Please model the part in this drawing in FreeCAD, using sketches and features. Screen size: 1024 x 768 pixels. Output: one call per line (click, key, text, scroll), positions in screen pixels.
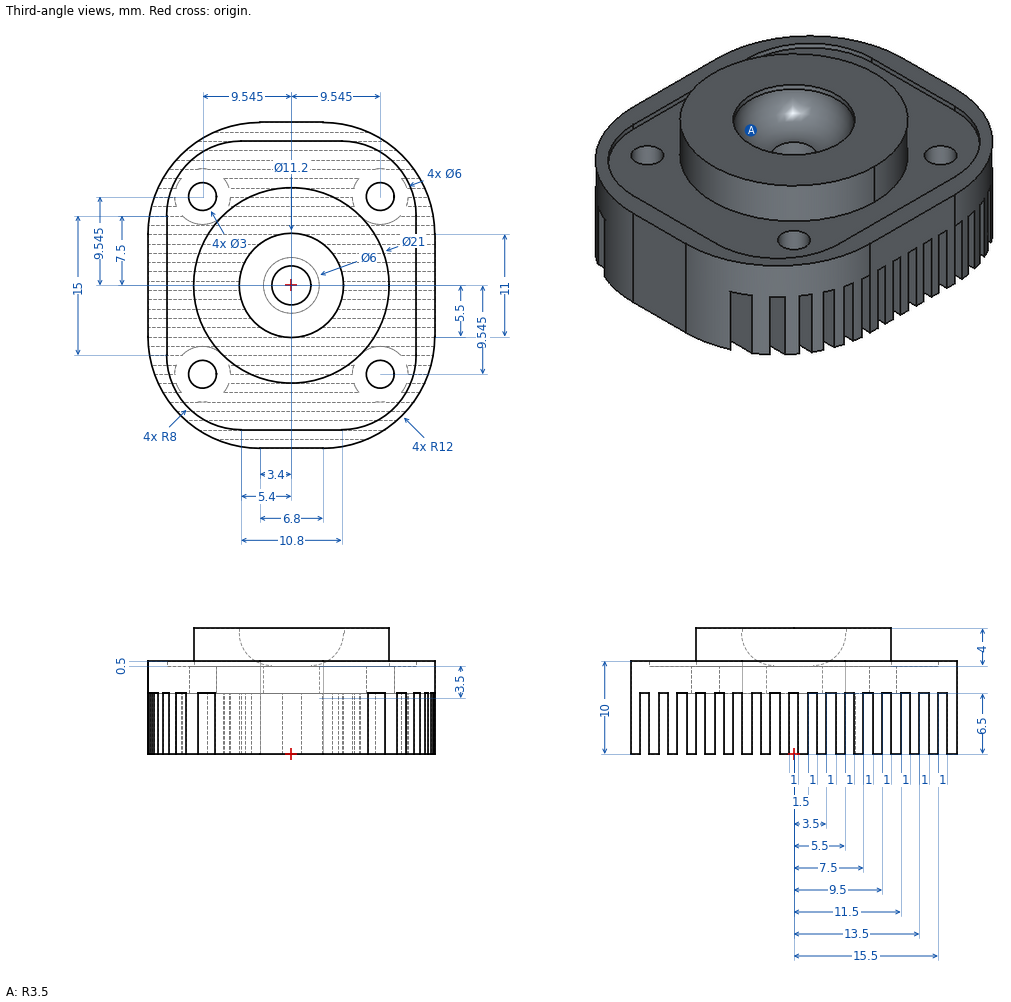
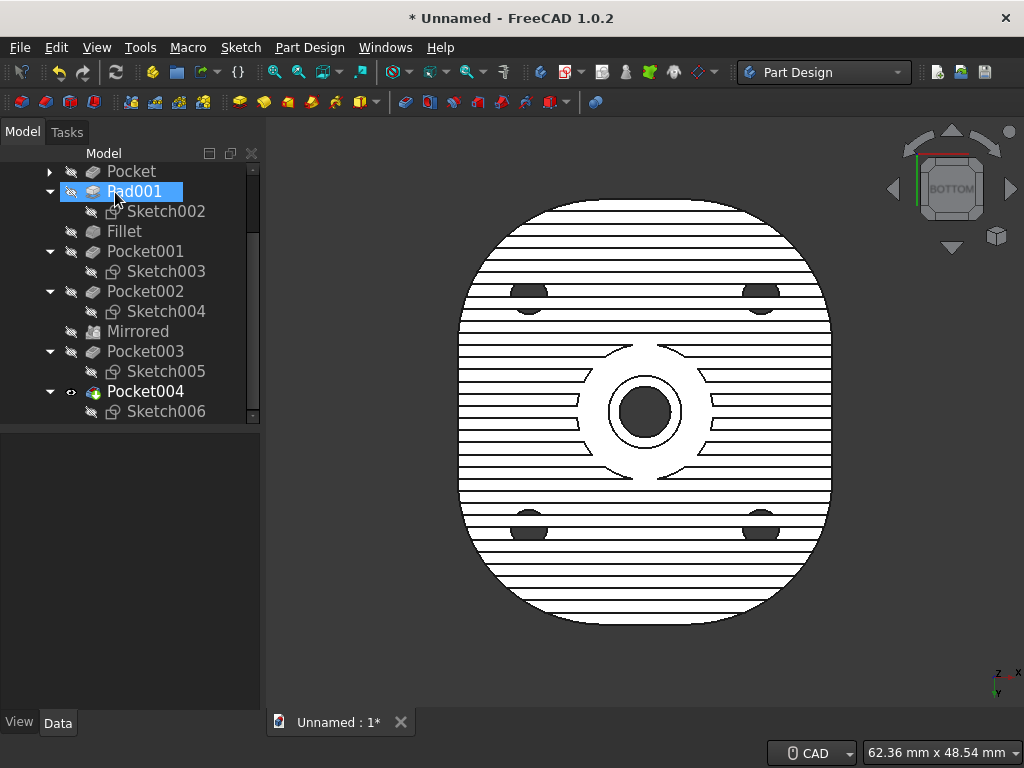
click(592, 411)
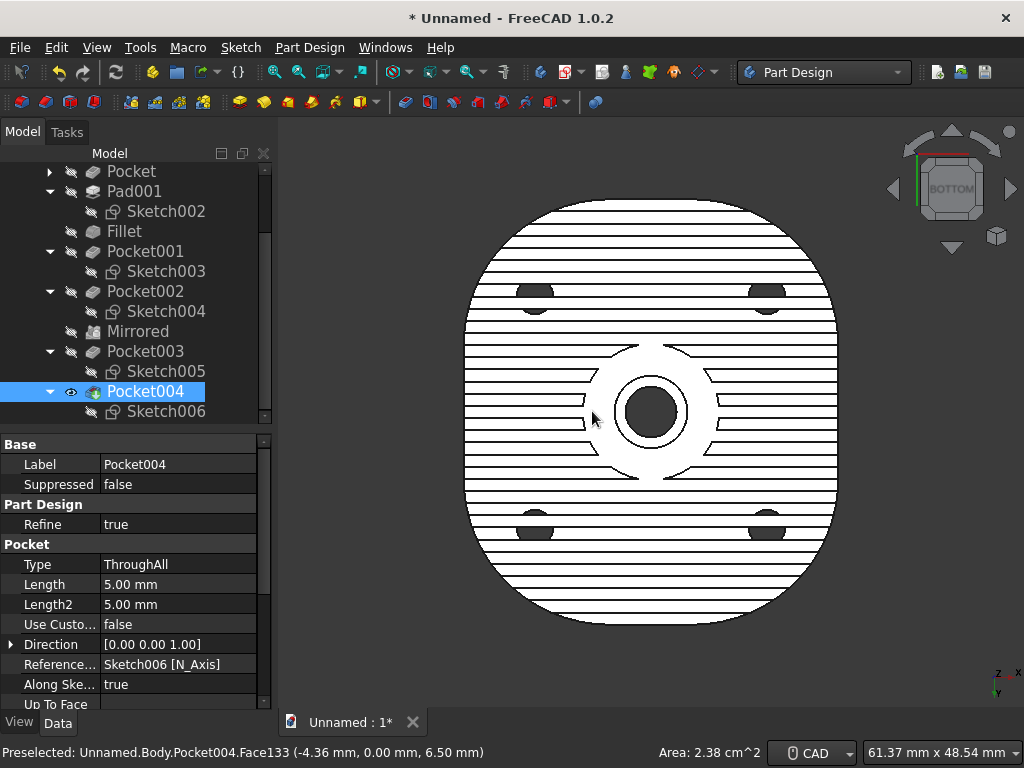
click(566, 72)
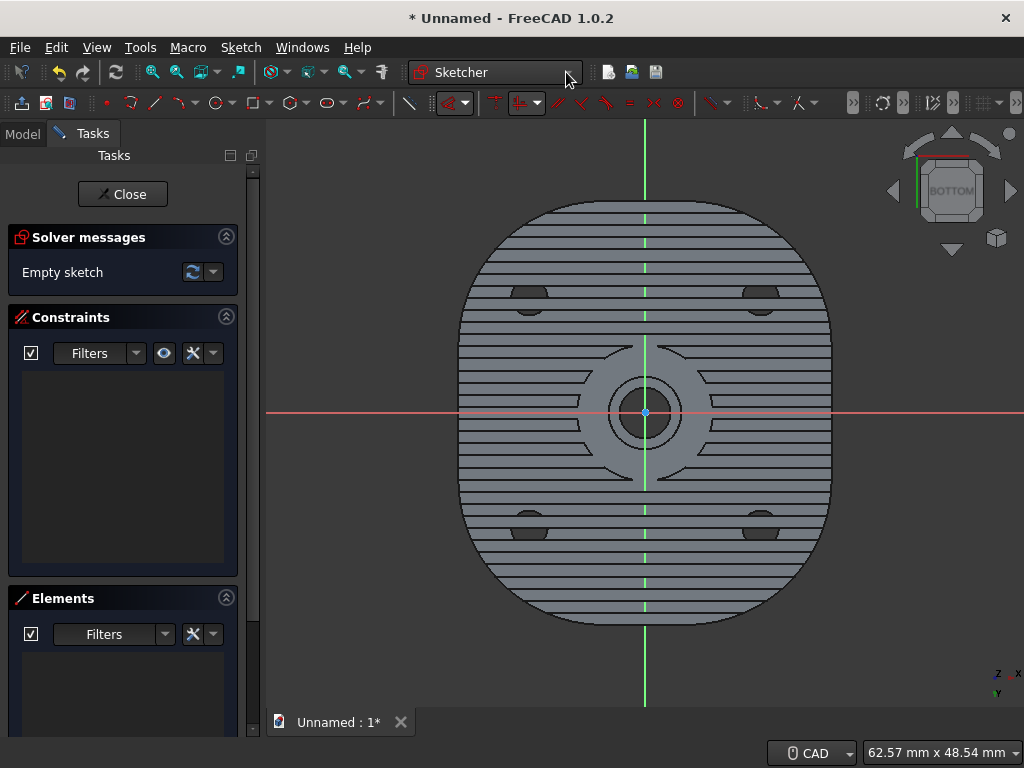
click(70, 104)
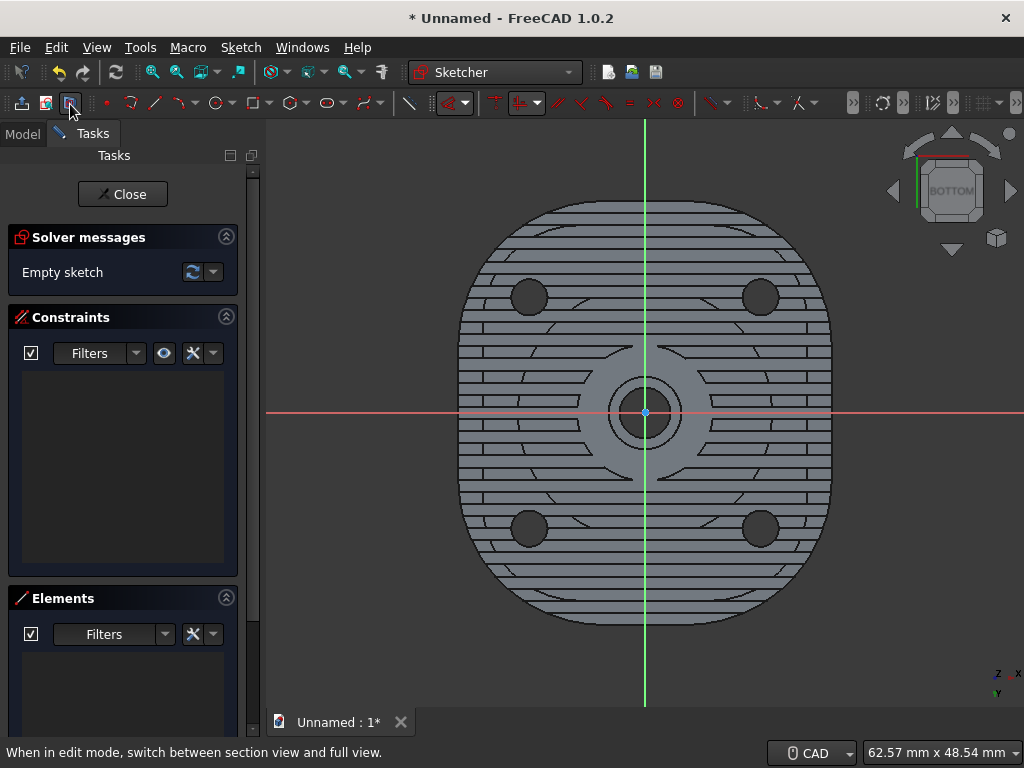
click(216, 104)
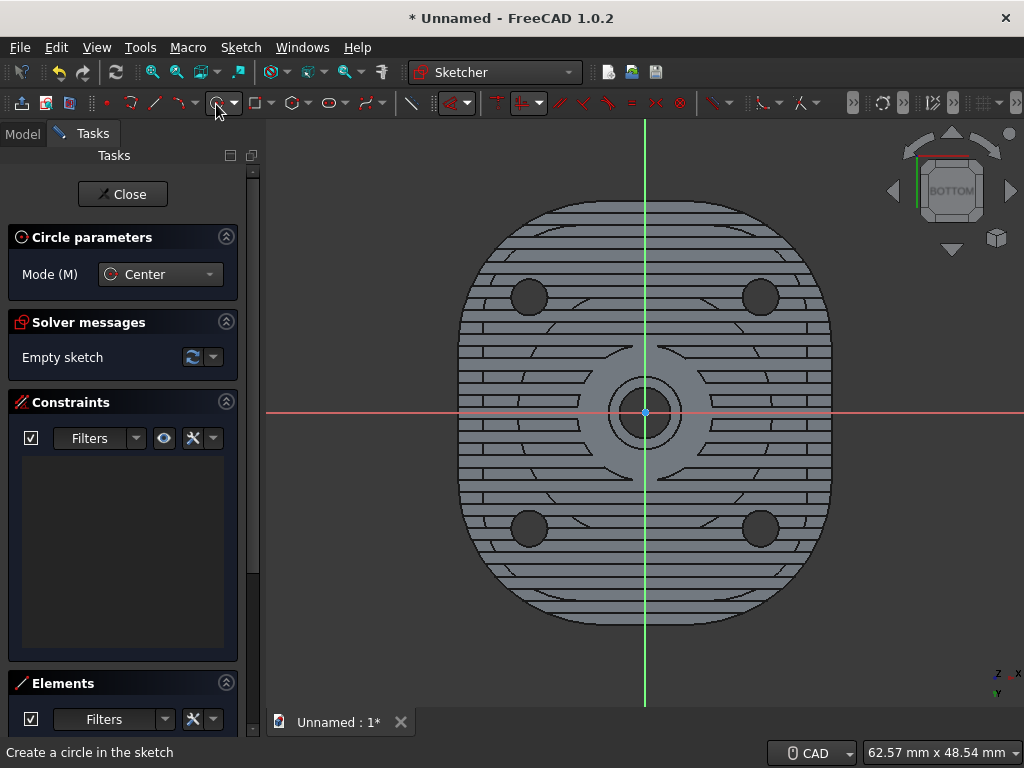
click(761, 529)
move(786, 503)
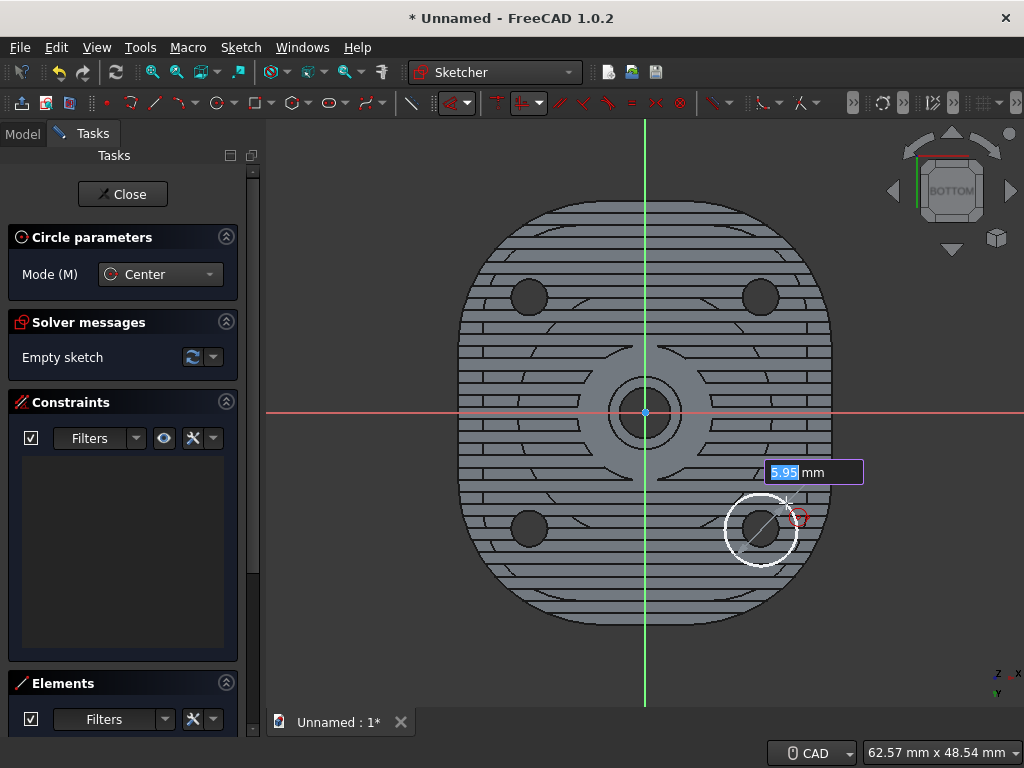
text(6)
key(Return)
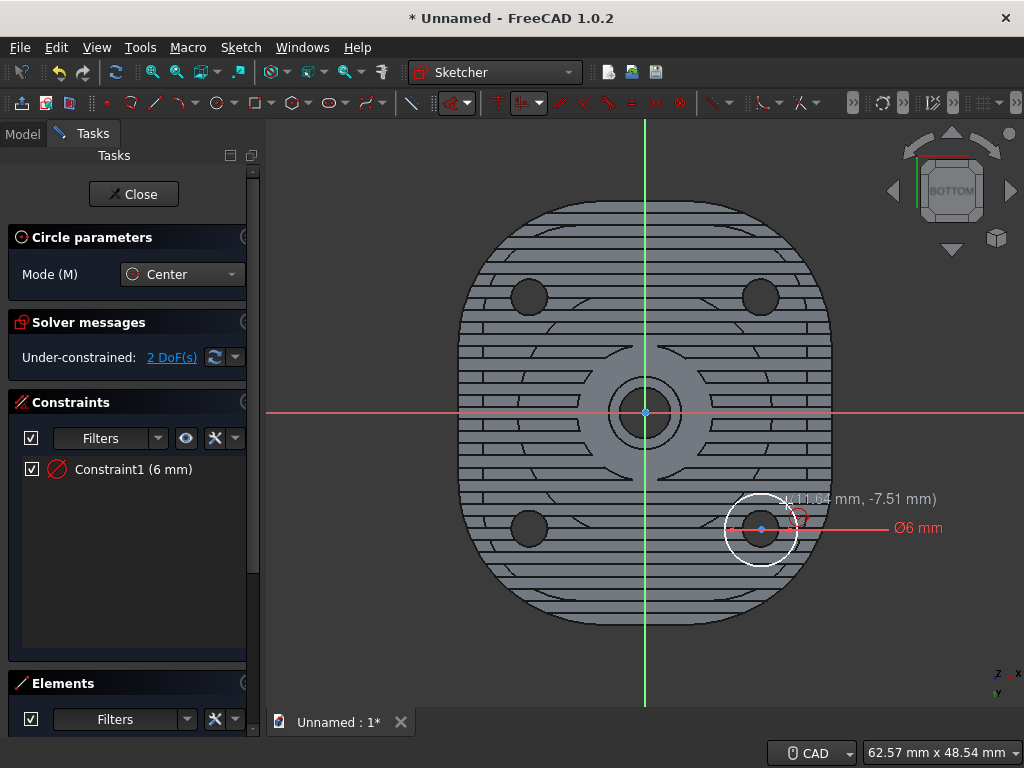
click(529, 529)
move(555, 503)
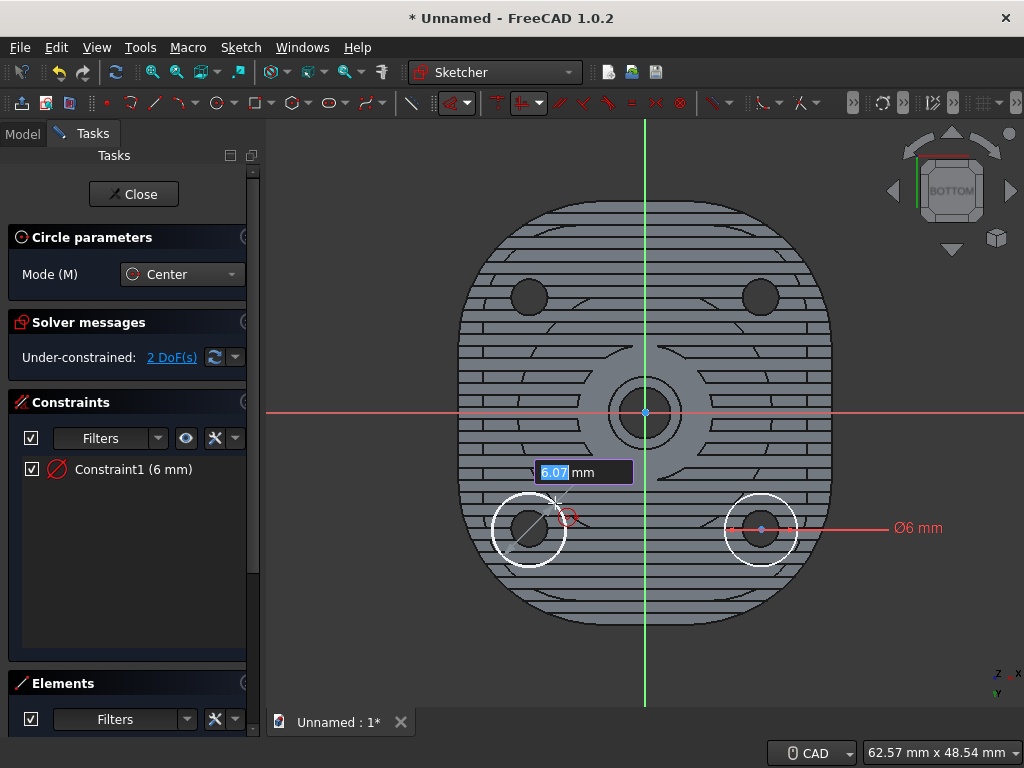
text(6)
key(Return)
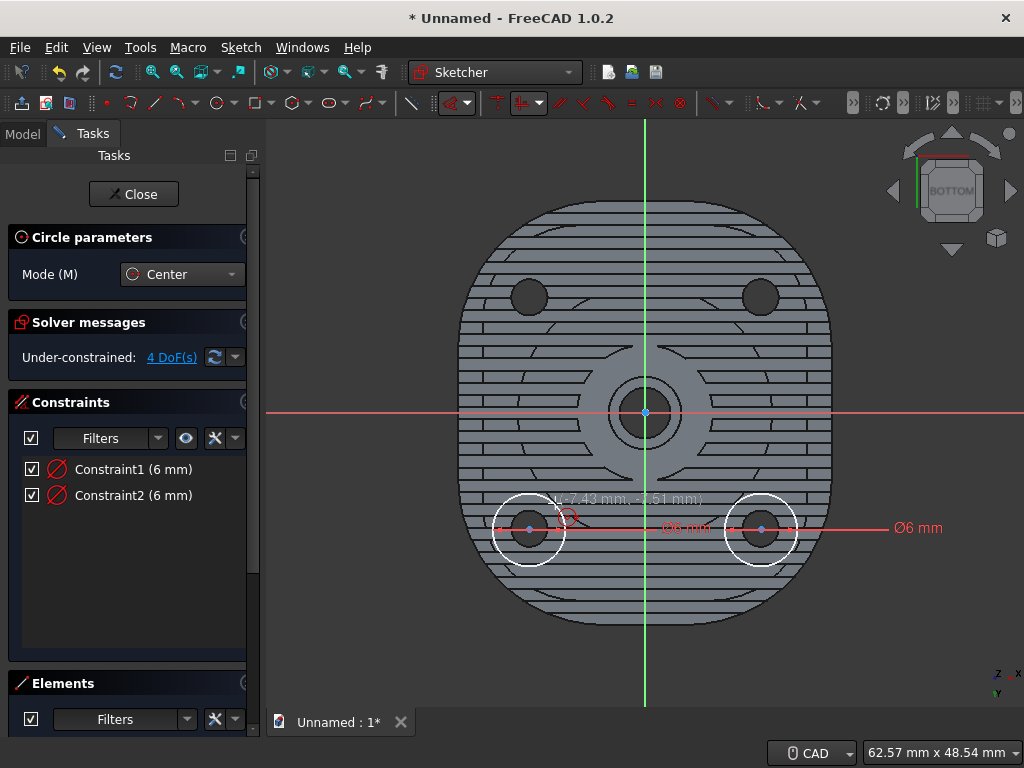
click(761, 297)
move(786, 272)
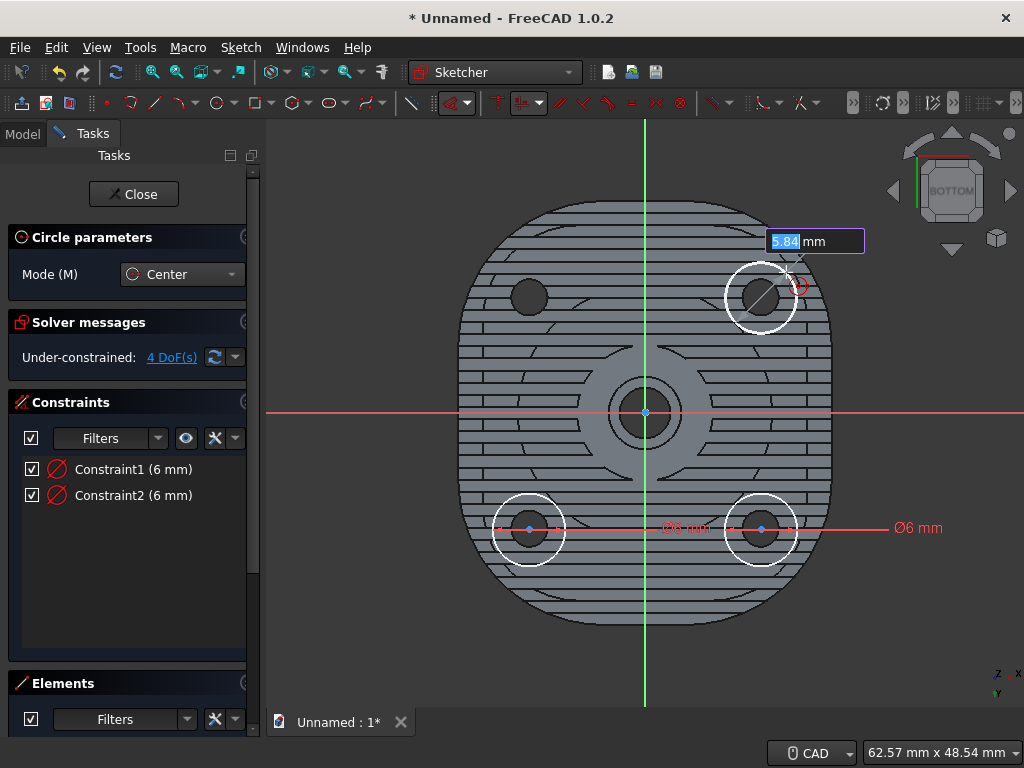
text(6)
key(Return)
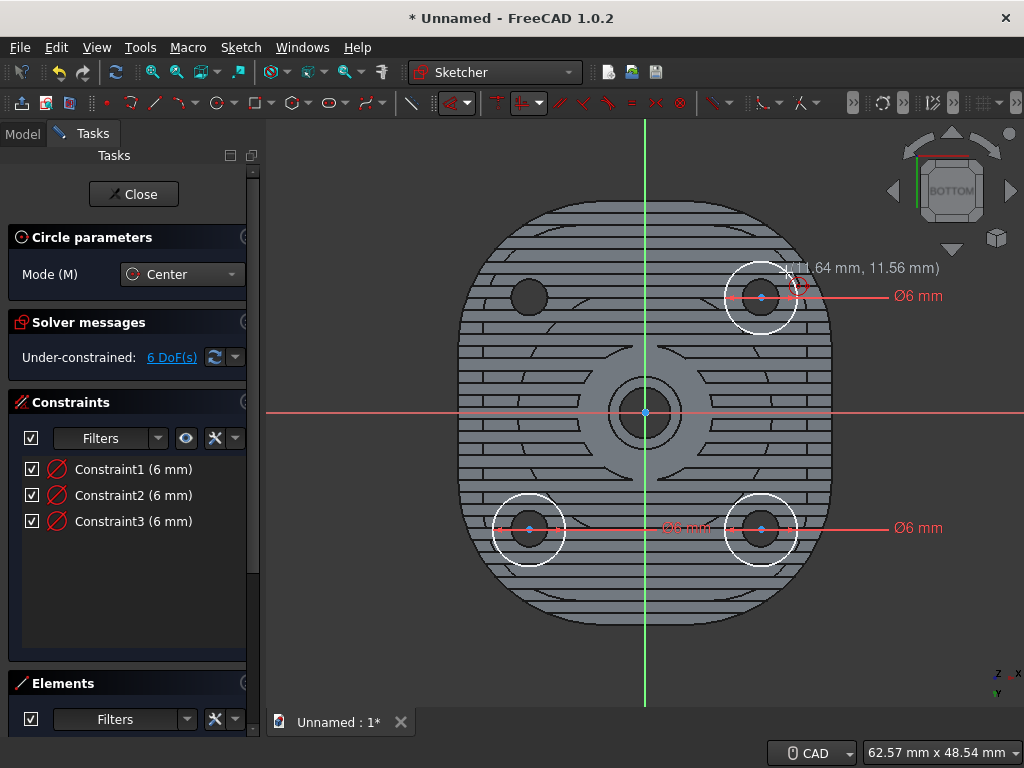
click(529, 297)
move(555, 272)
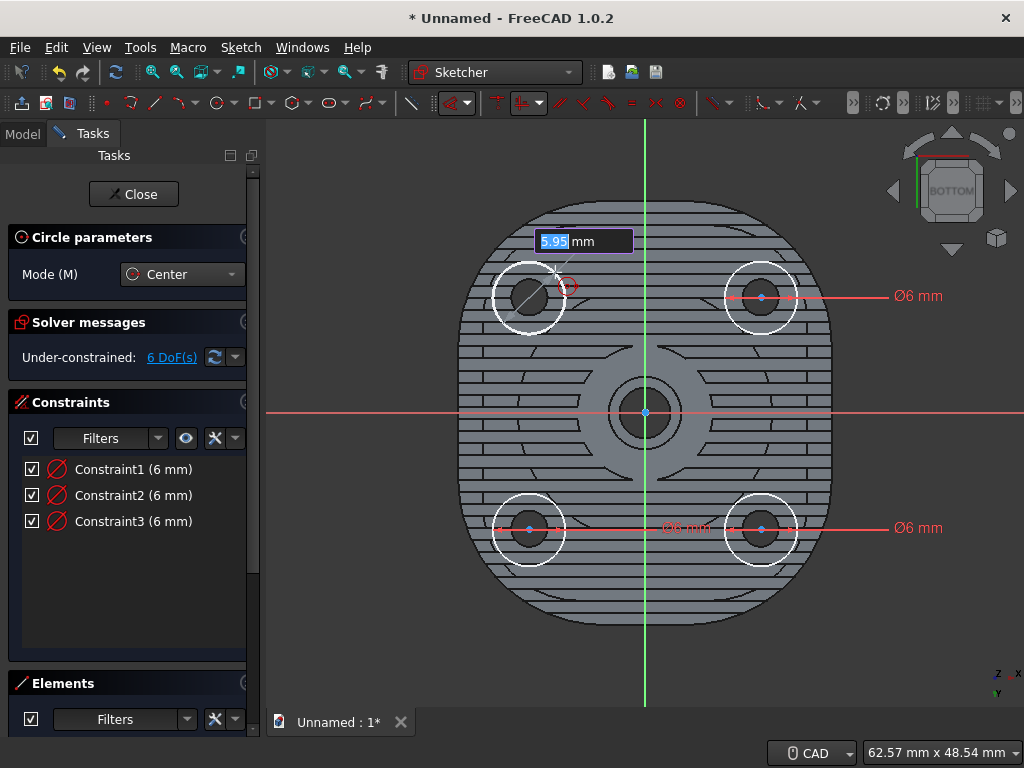
text(6)
key(Return)
key(Escape)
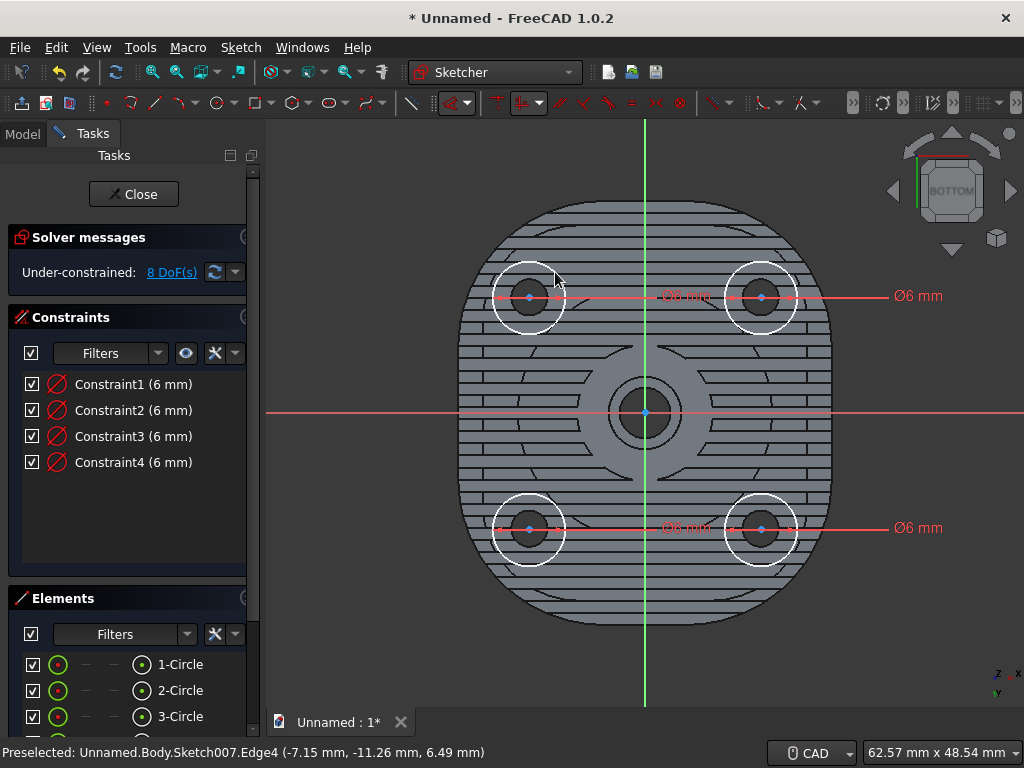
click(761, 530)